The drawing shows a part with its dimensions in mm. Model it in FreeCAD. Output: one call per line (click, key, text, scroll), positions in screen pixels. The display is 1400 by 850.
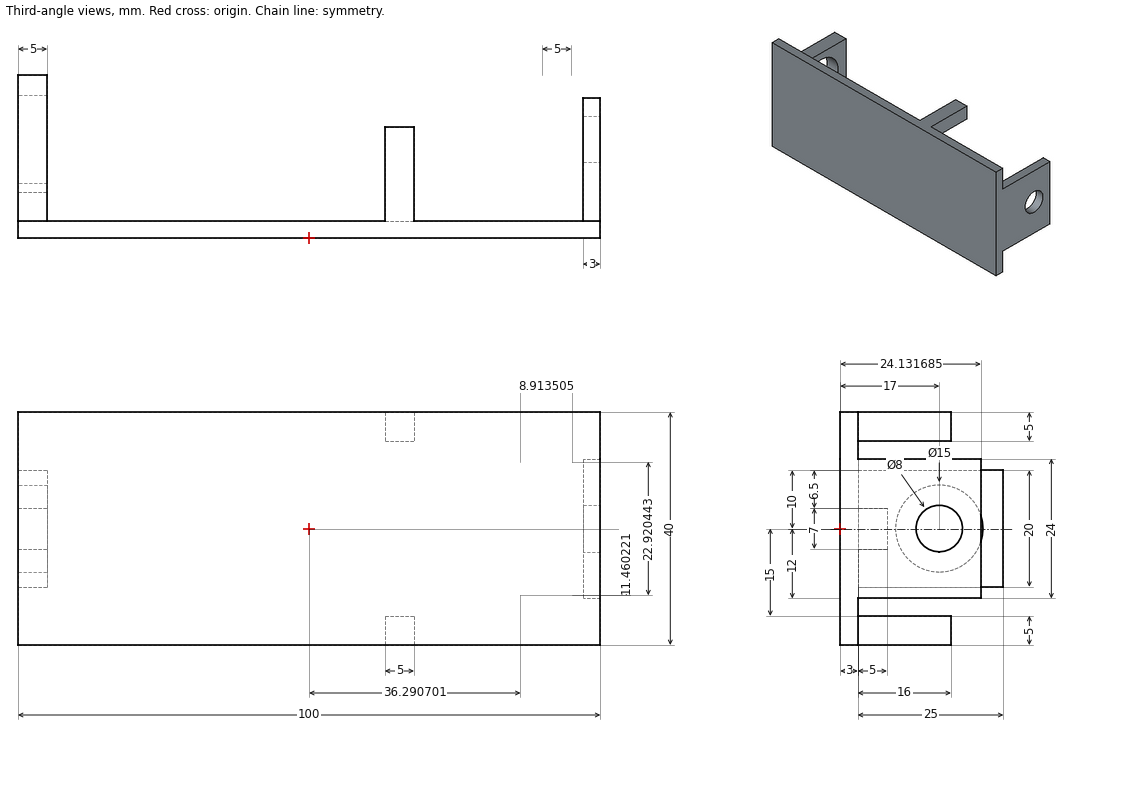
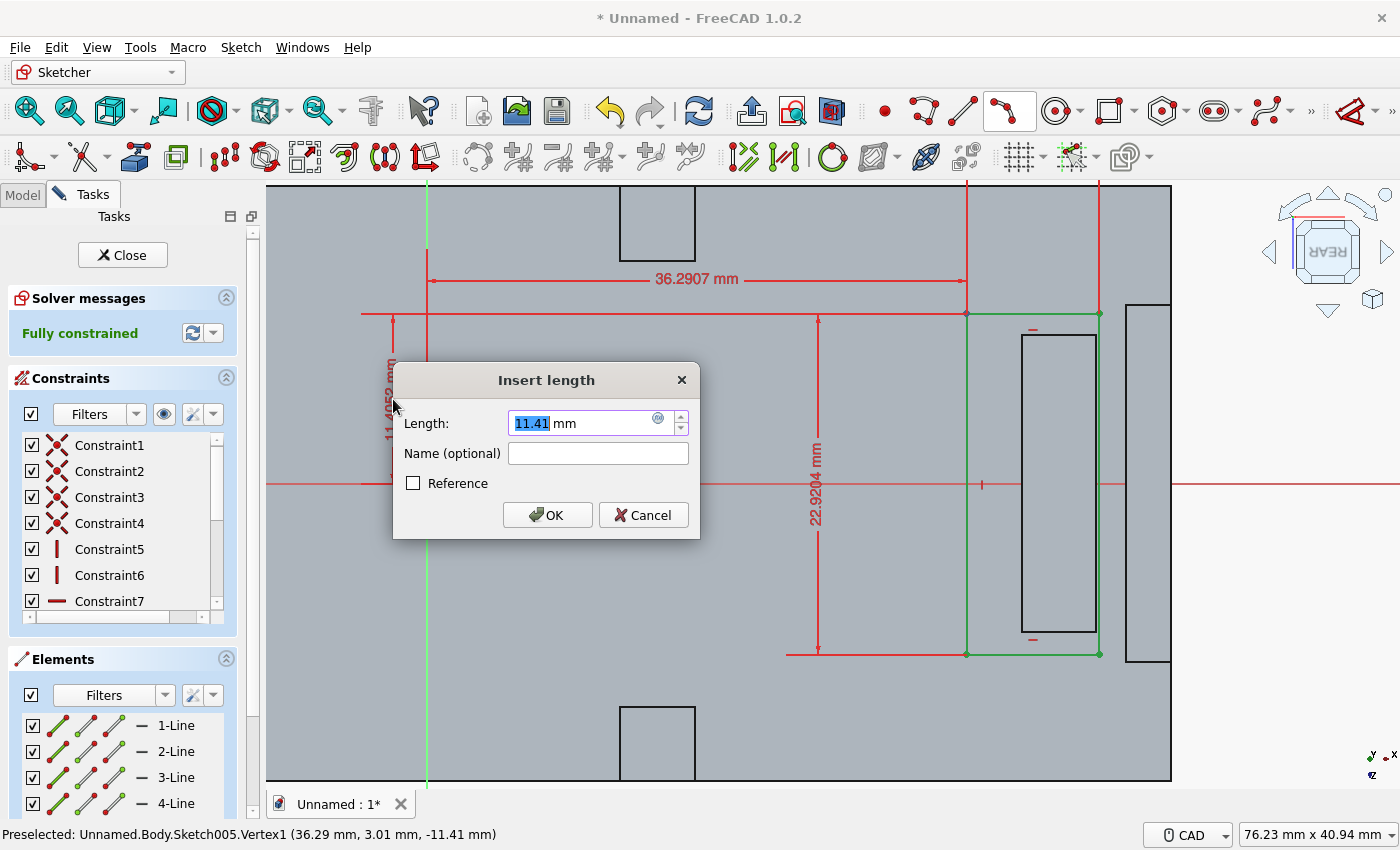
text(11.460221)
key(Return)
key(Escape)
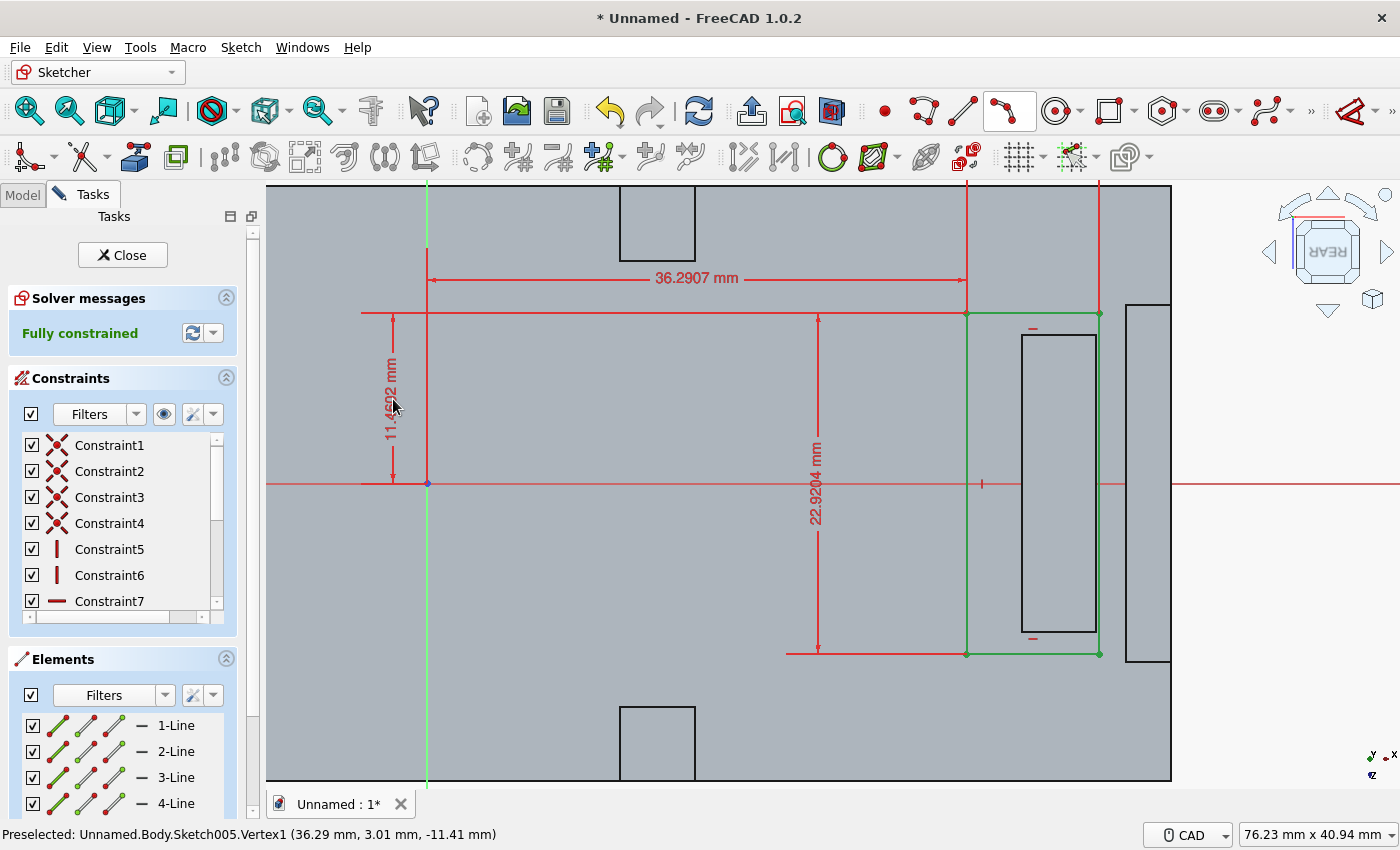
click(123, 255)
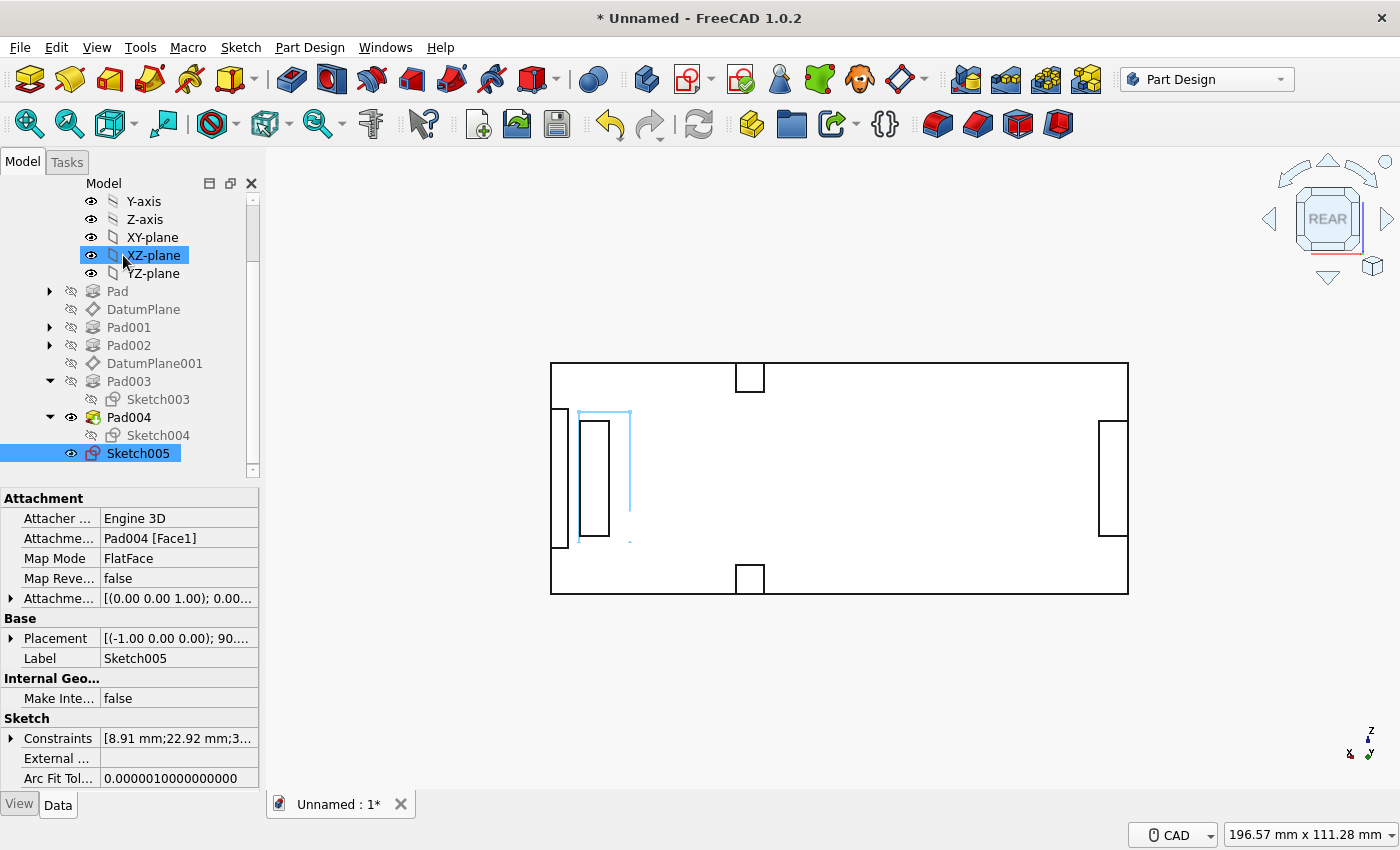
click(292, 80)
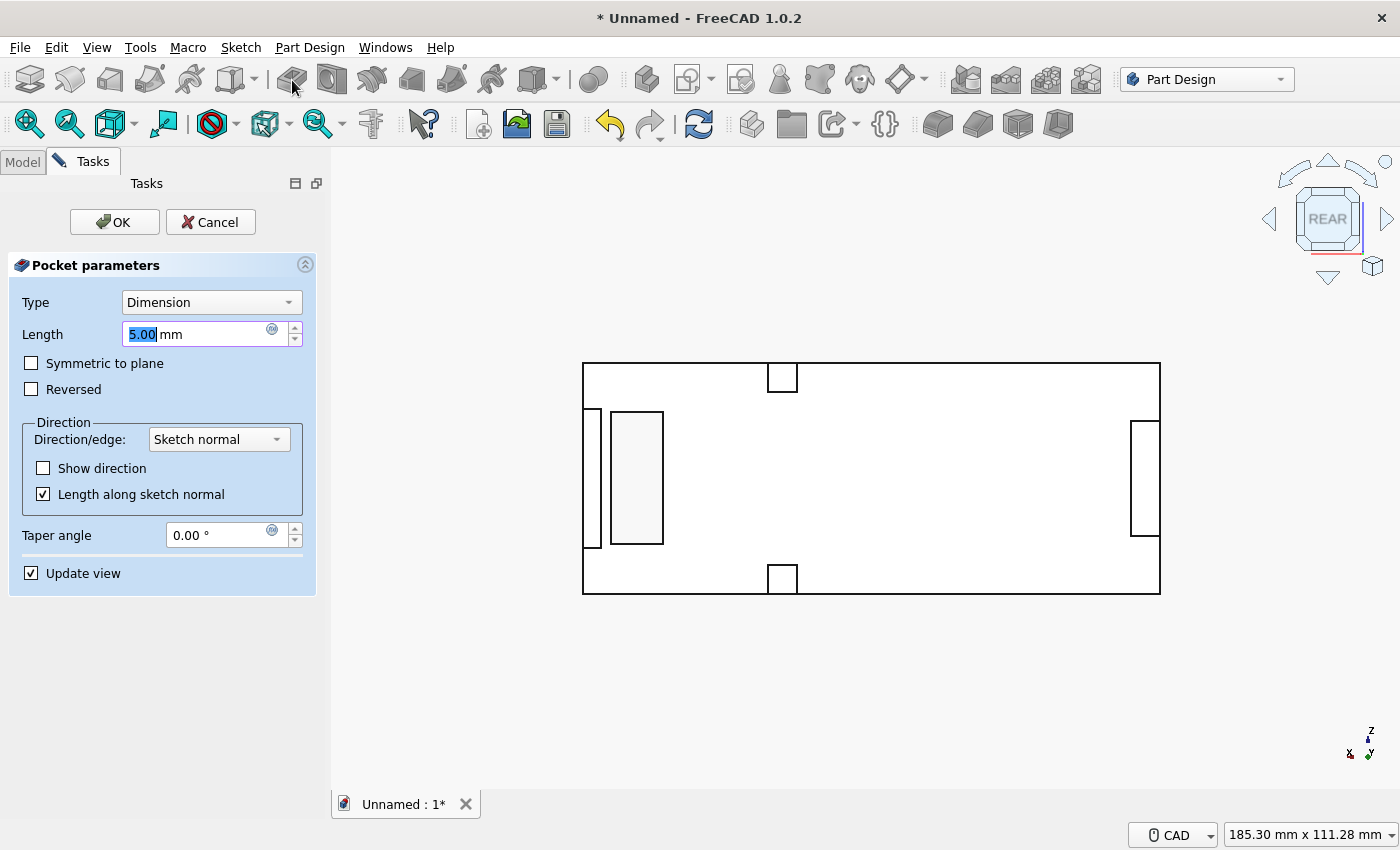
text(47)
key(Tab)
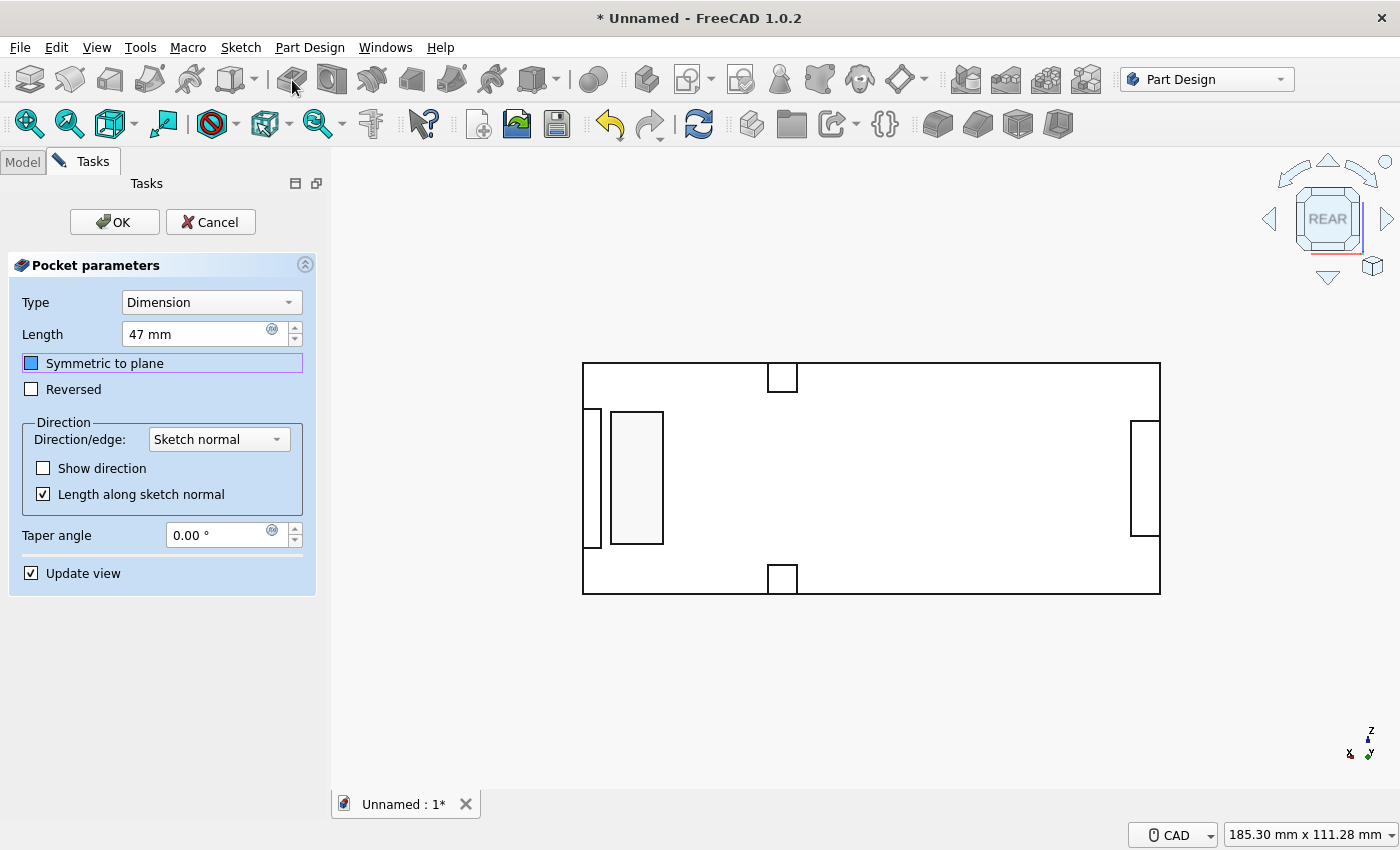
click(30, 389)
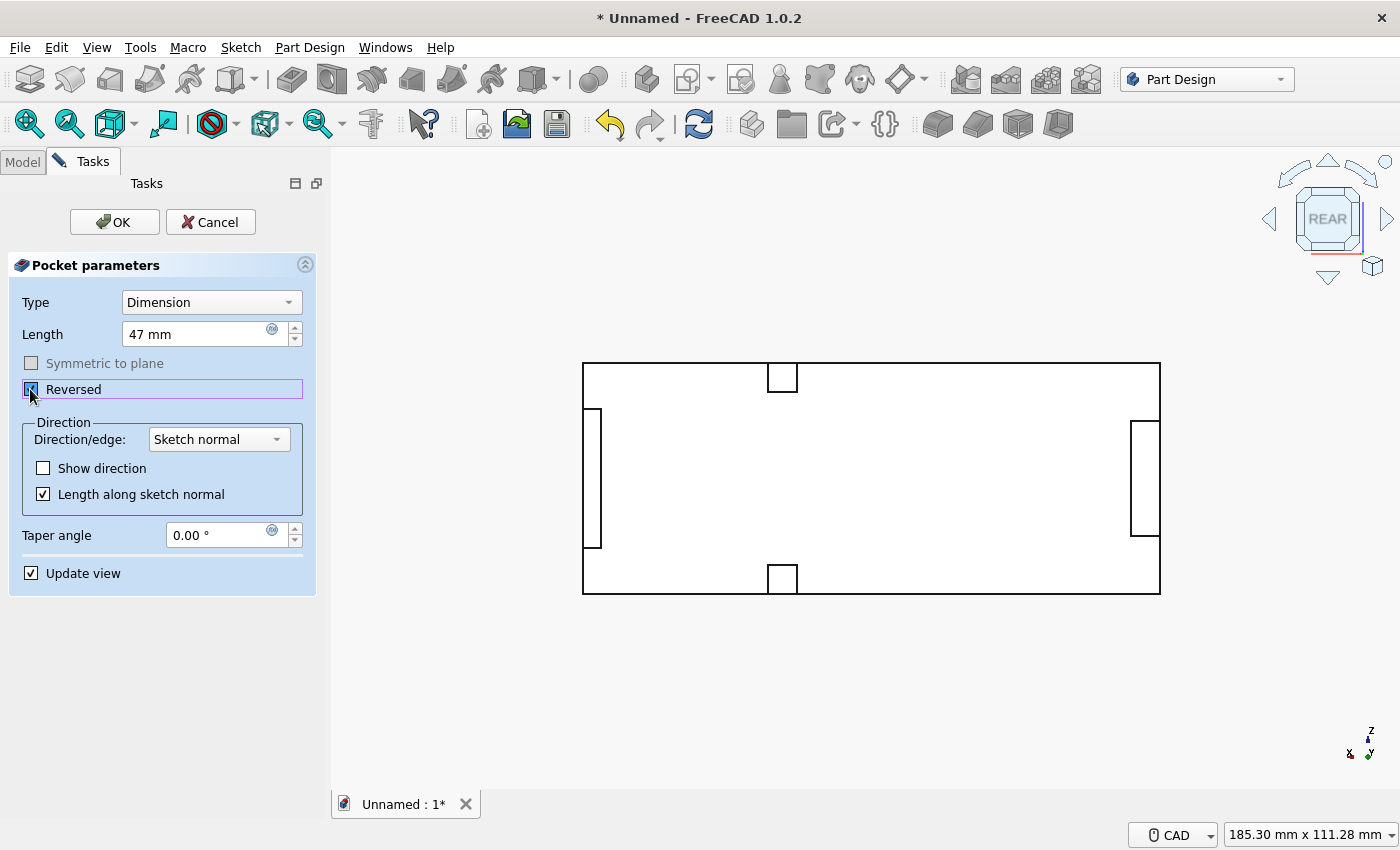
click(115, 222)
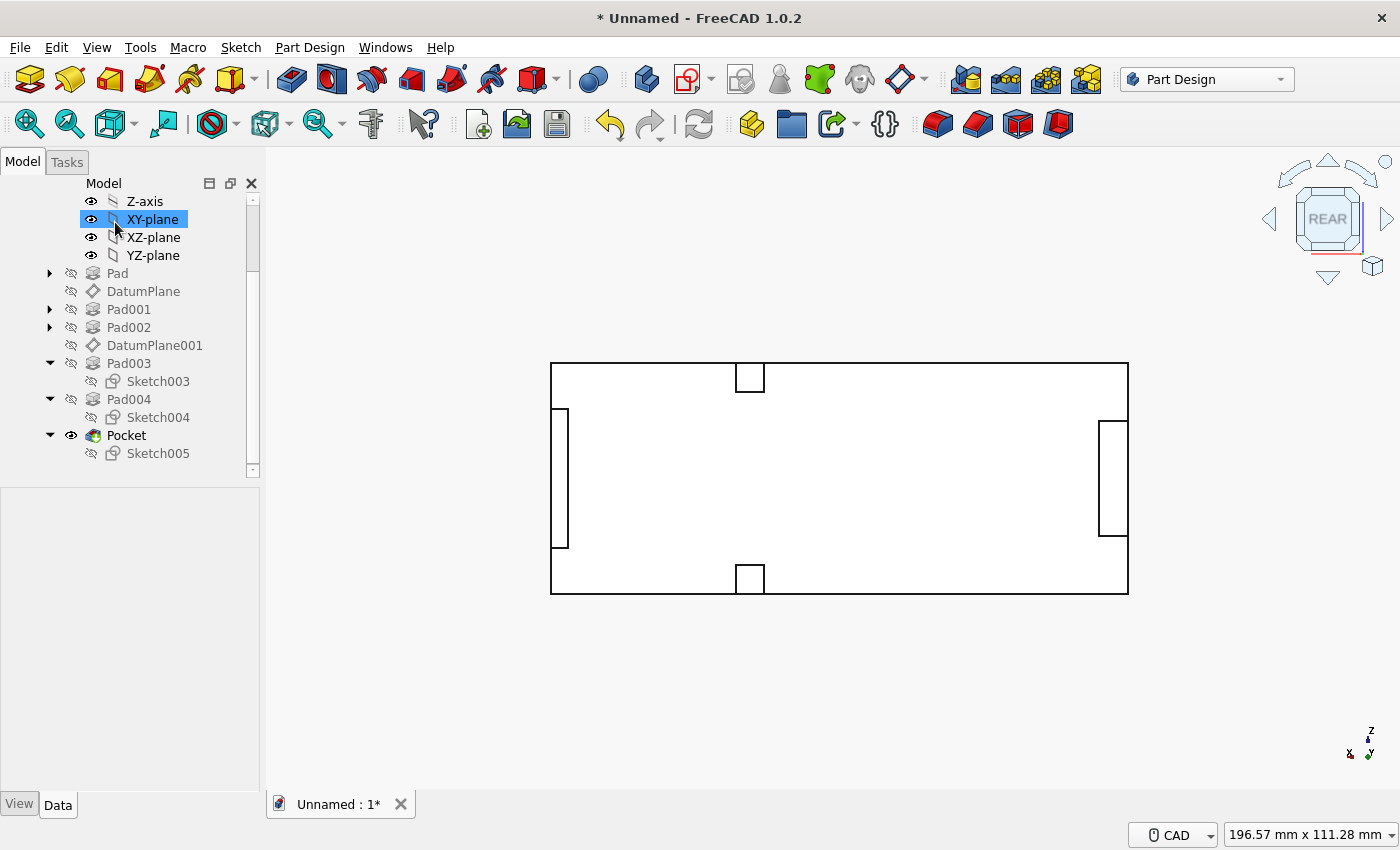
key(0)